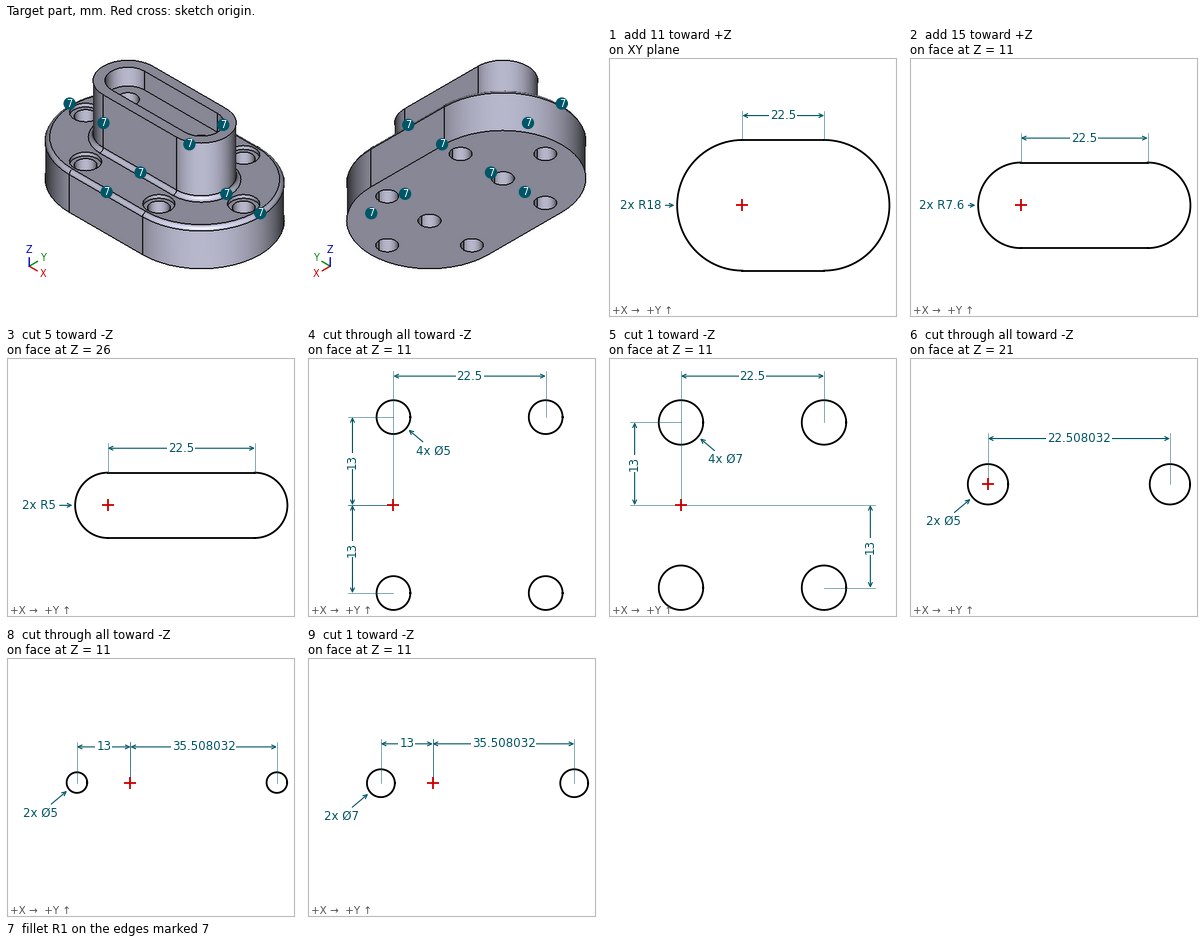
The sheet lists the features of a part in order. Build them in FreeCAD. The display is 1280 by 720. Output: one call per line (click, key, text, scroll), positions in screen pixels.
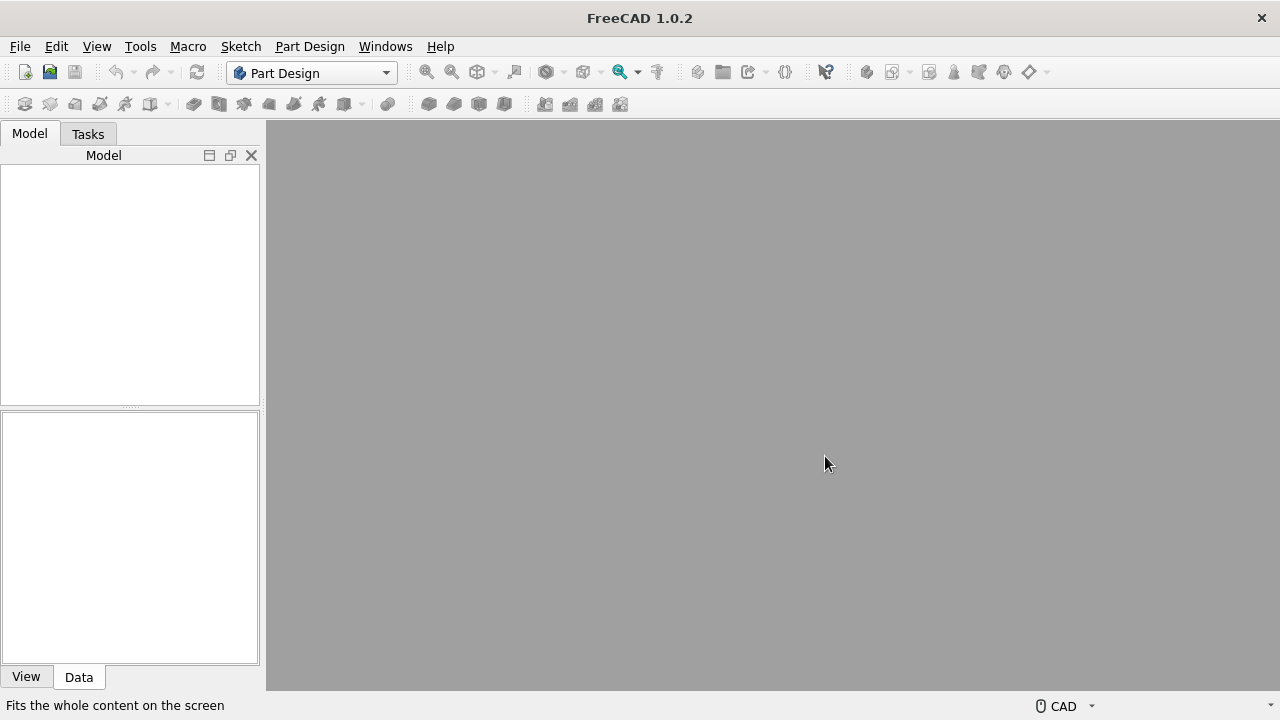
click(25, 72)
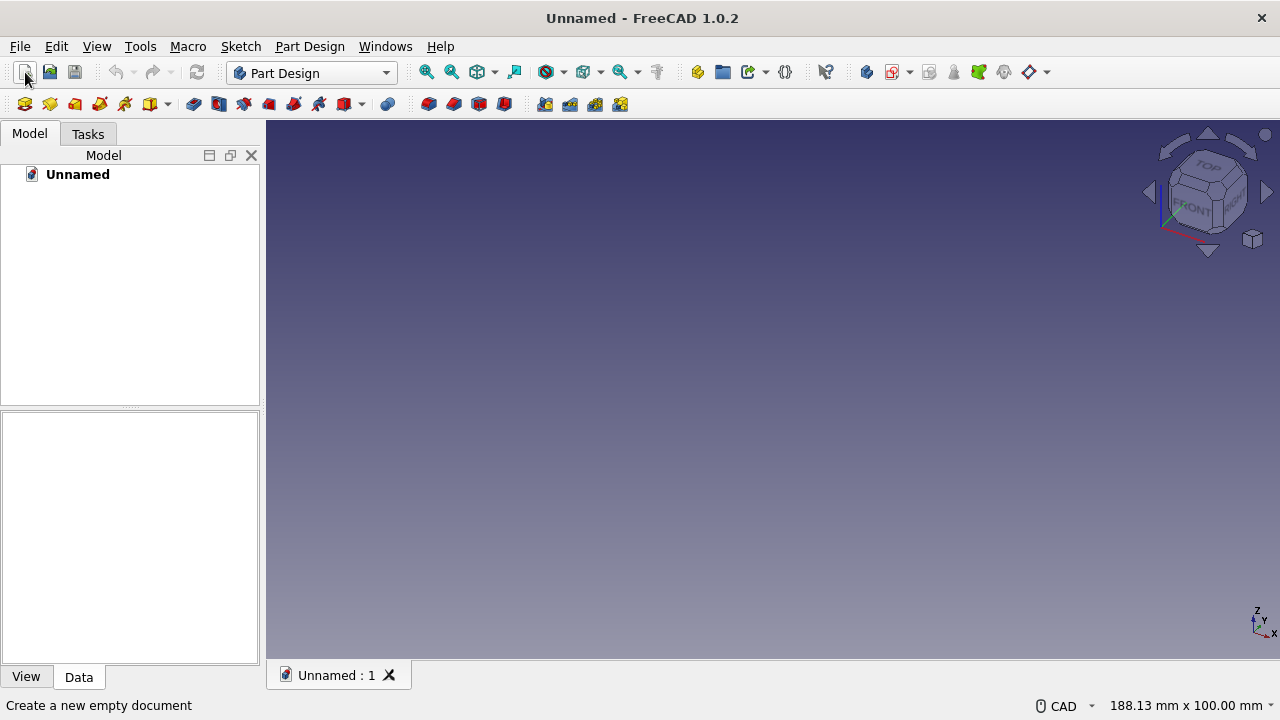
click(892, 72)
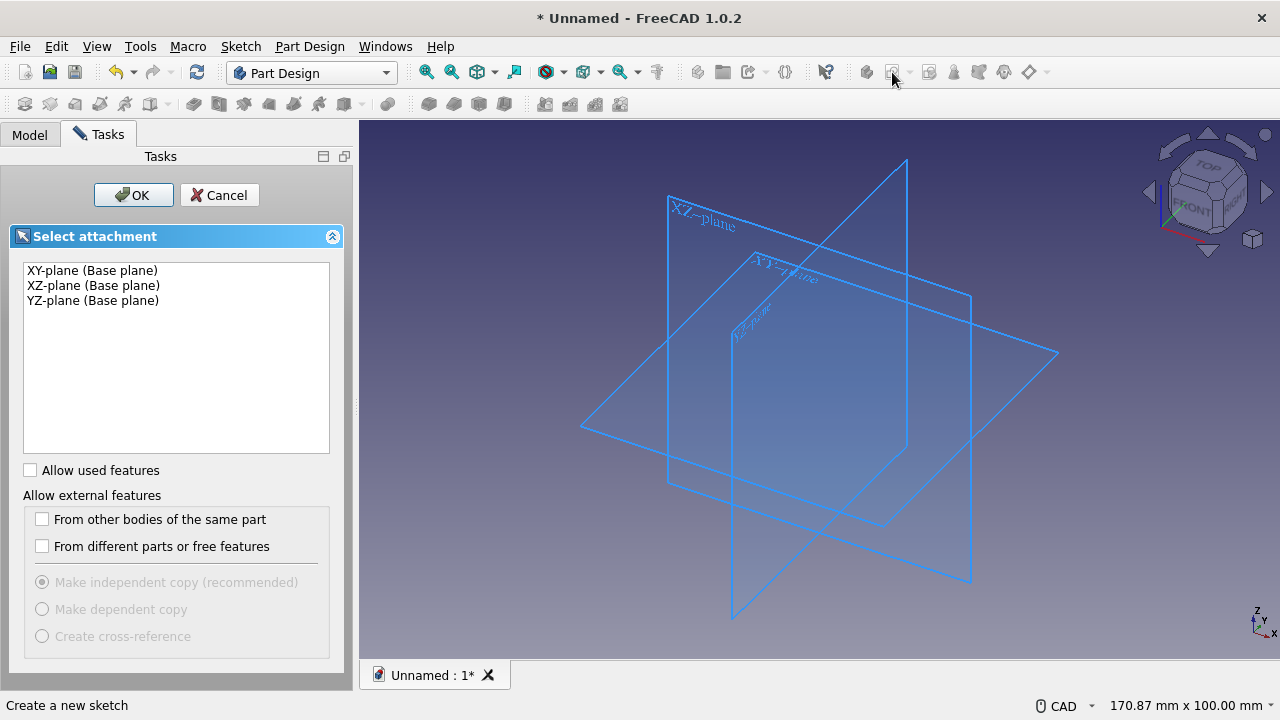
click(84, 270)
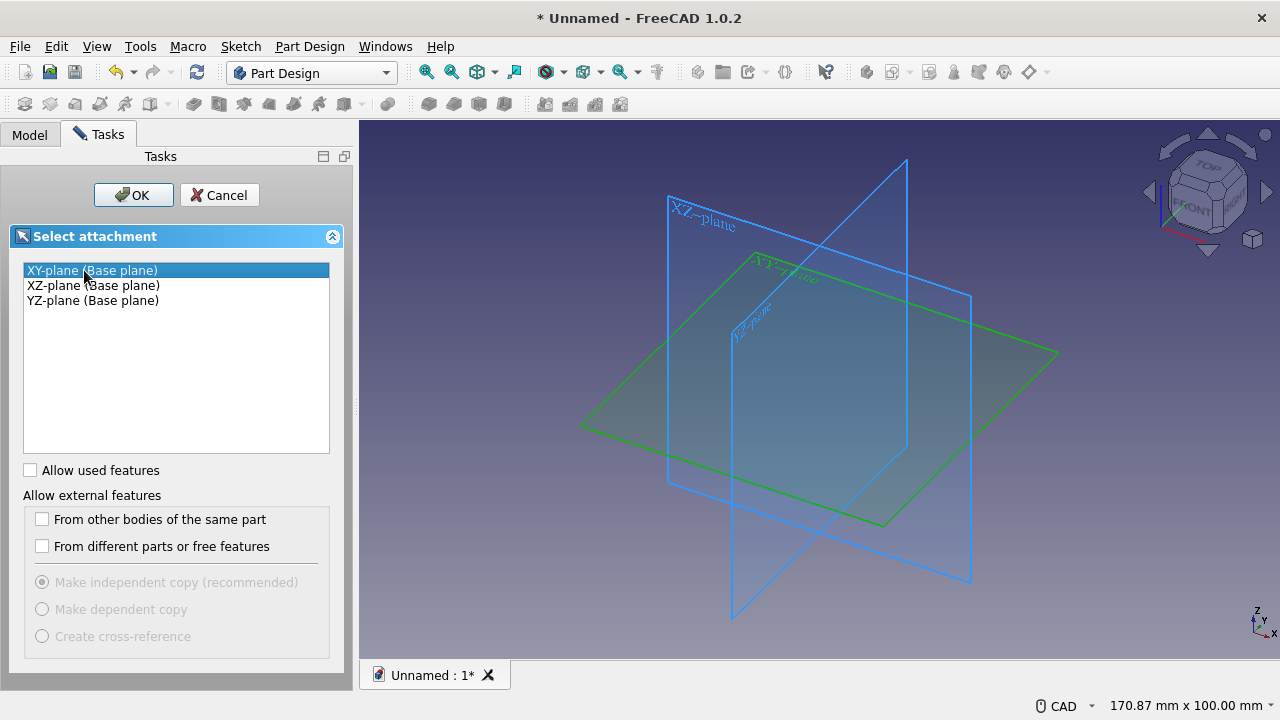
click(134, 195)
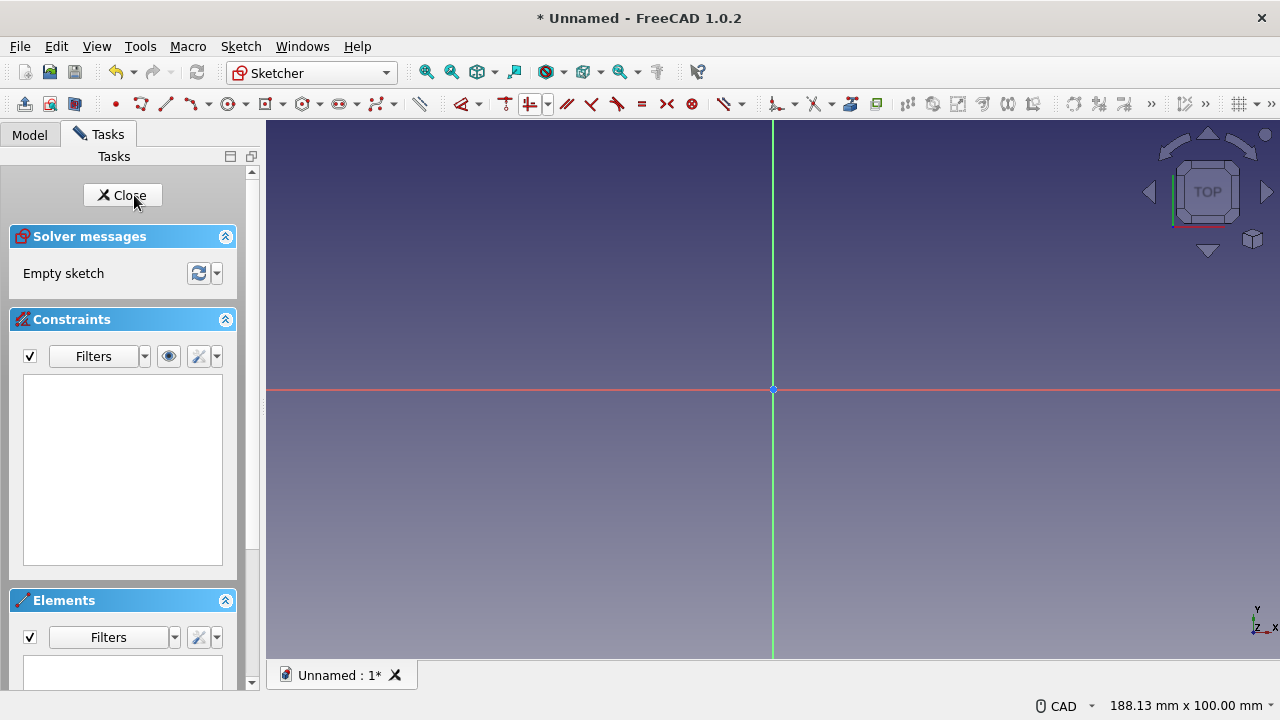
scroll(991, 389, up, 3)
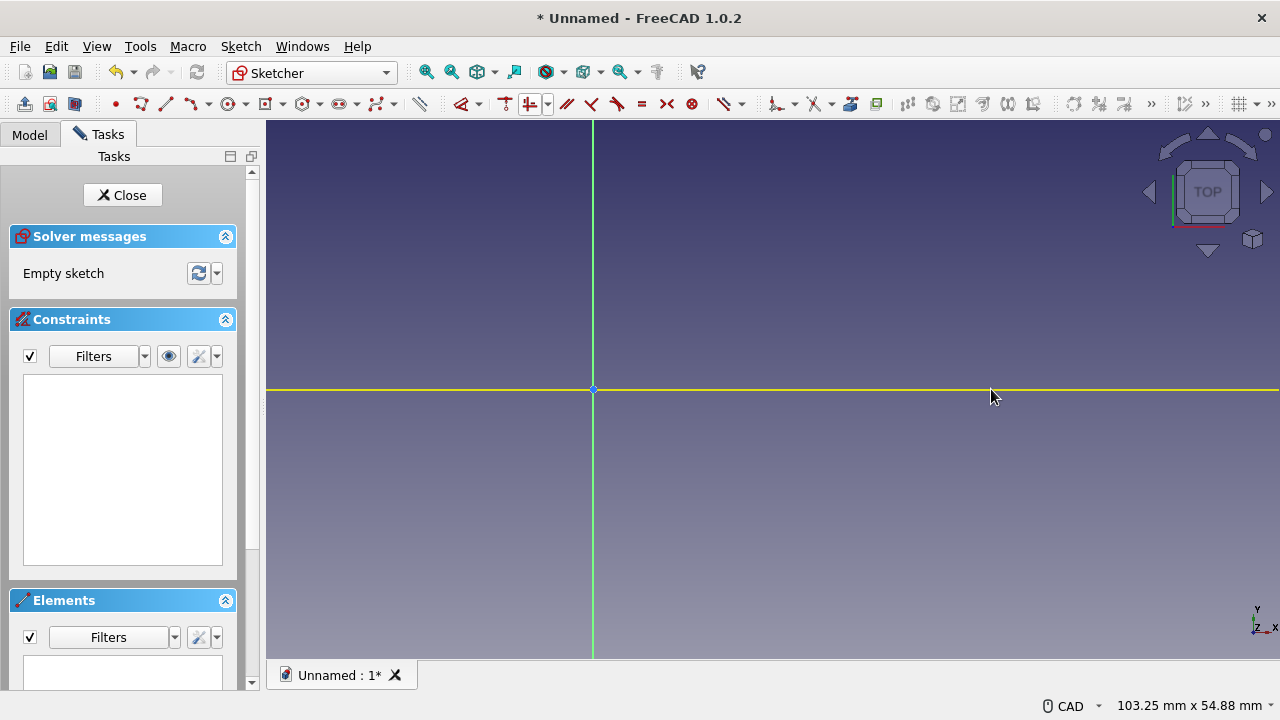
key(g)
key(s)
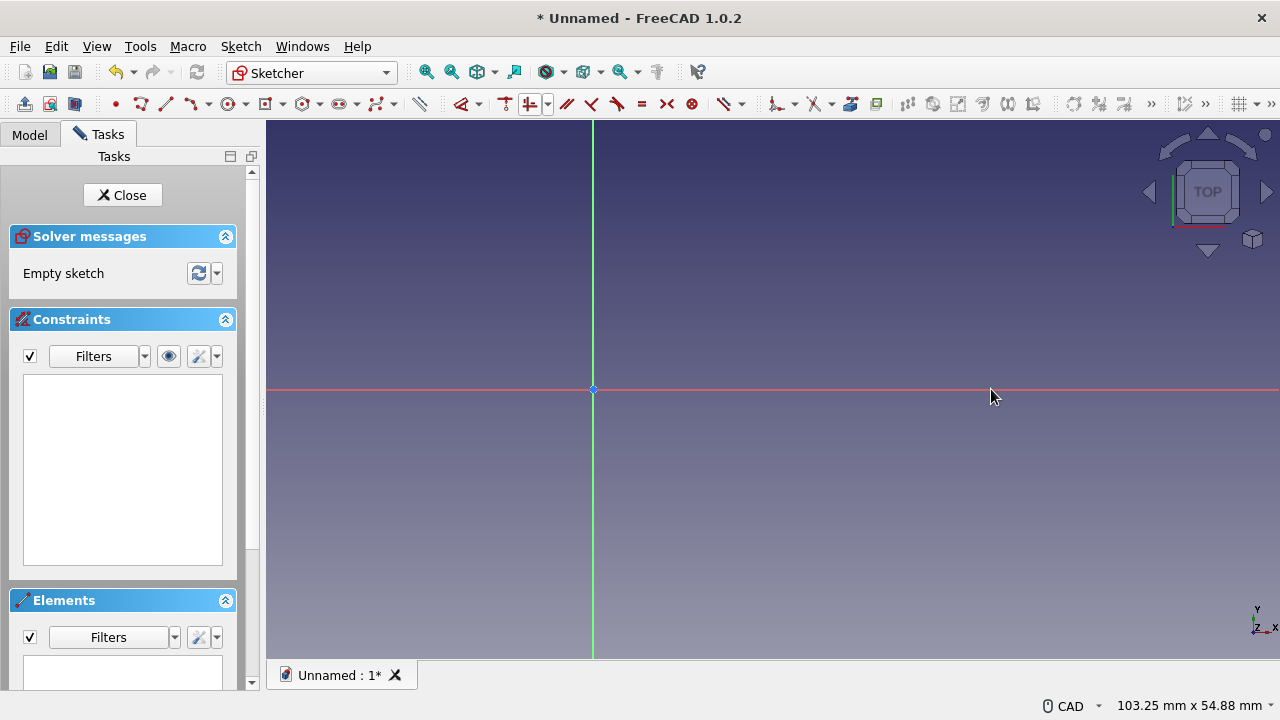
click(593, 390)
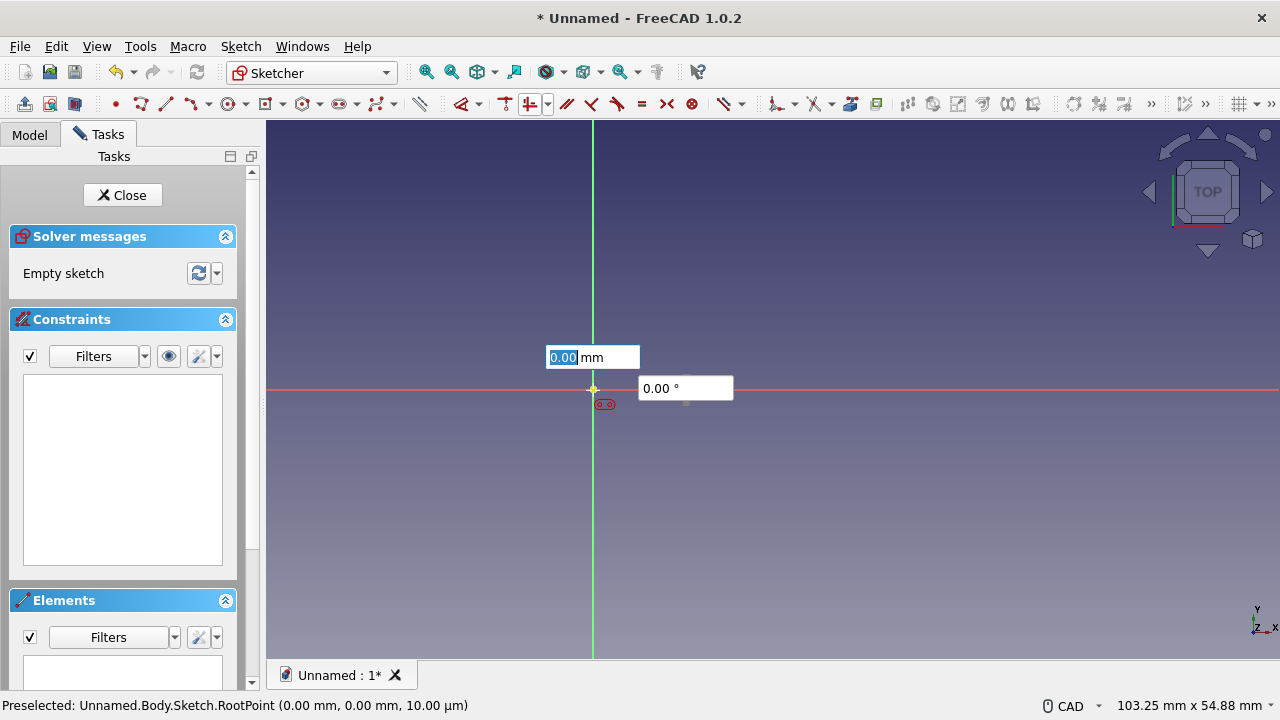
click(814, 380)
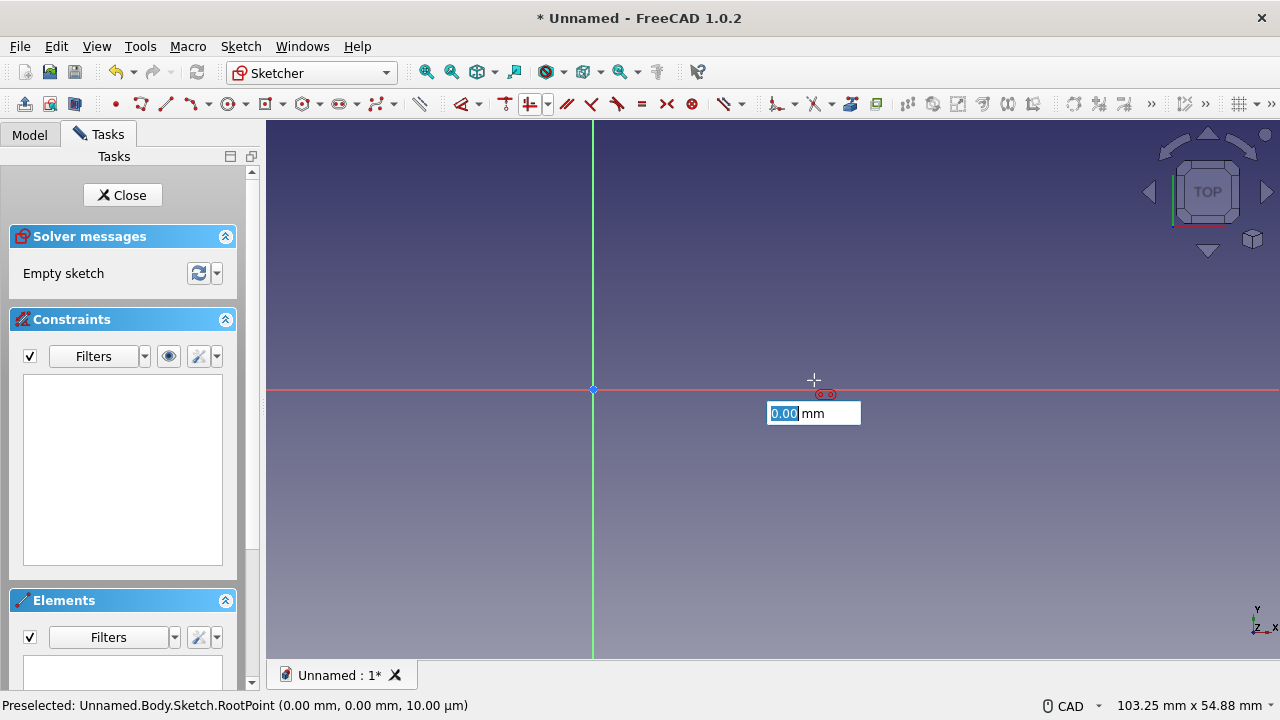
click(704, 213)
key(Escape)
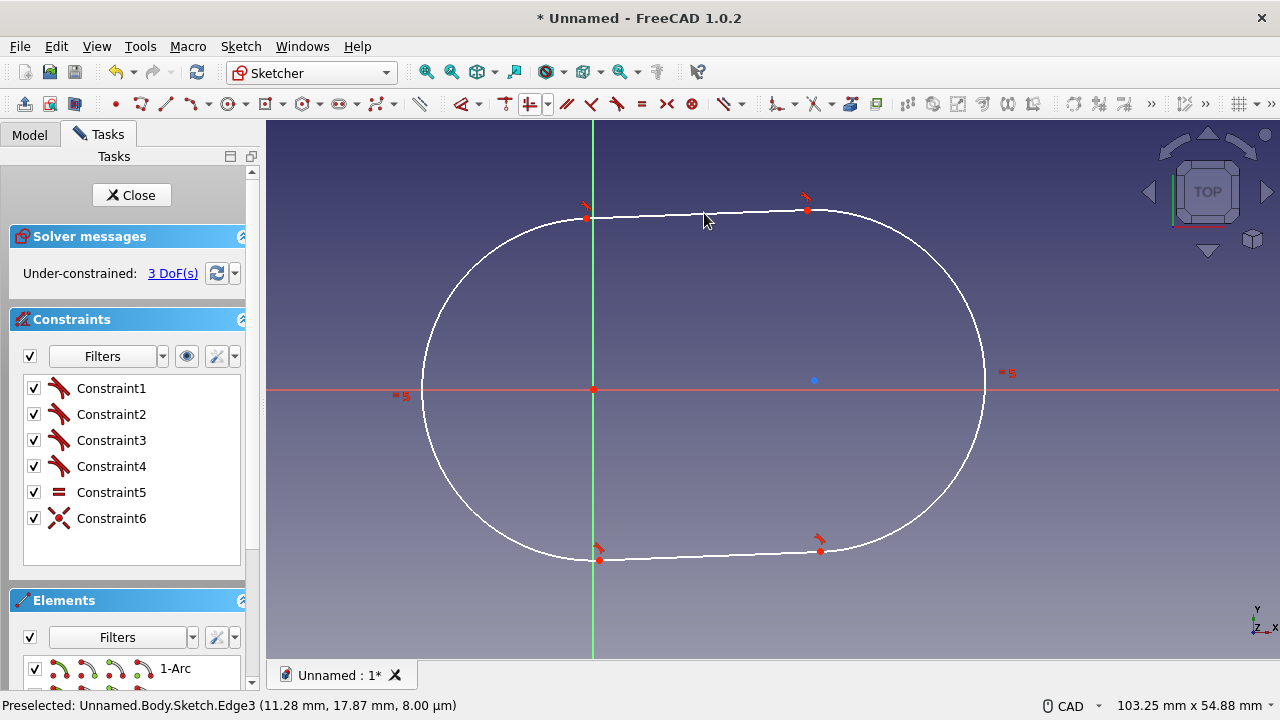
click(653, 216)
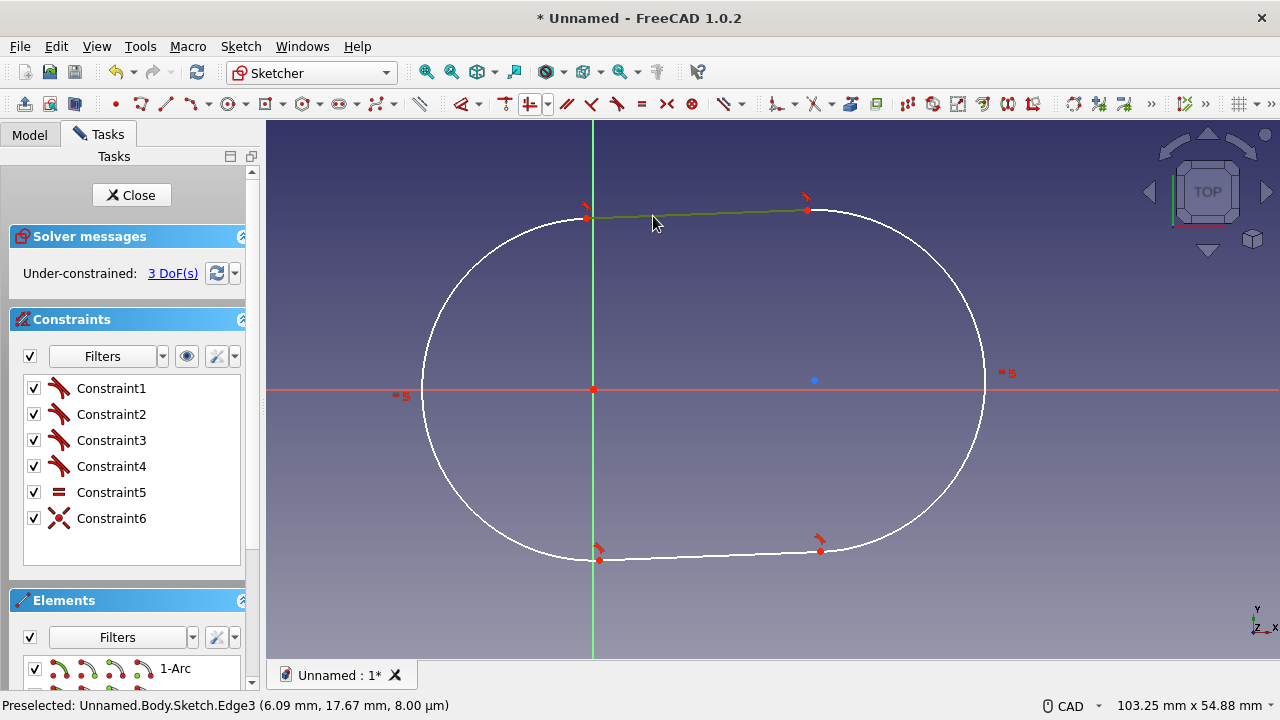
key(h)